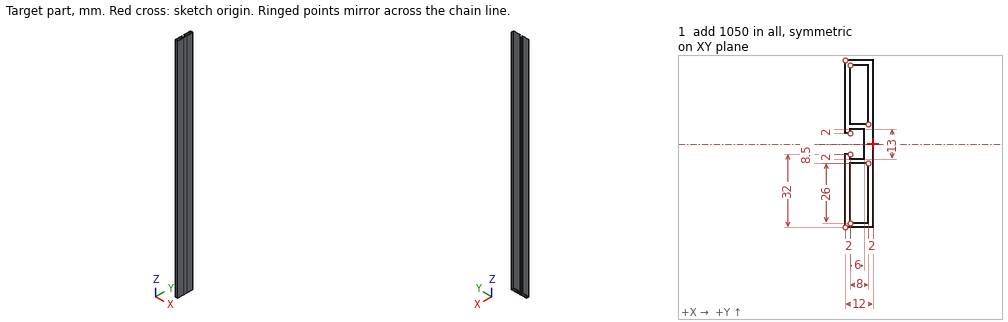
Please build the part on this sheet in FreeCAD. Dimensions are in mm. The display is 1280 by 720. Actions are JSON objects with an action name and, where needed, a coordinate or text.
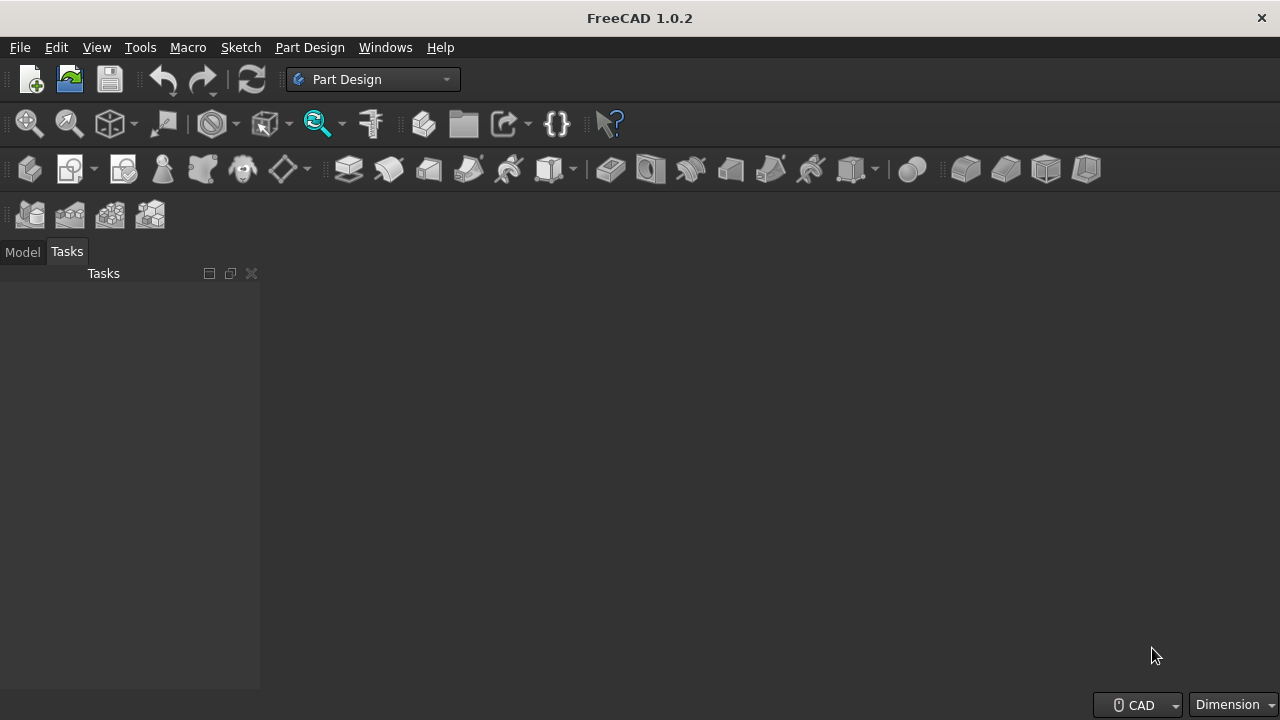
{"action": "left_click", "coordinate": [30, 80]}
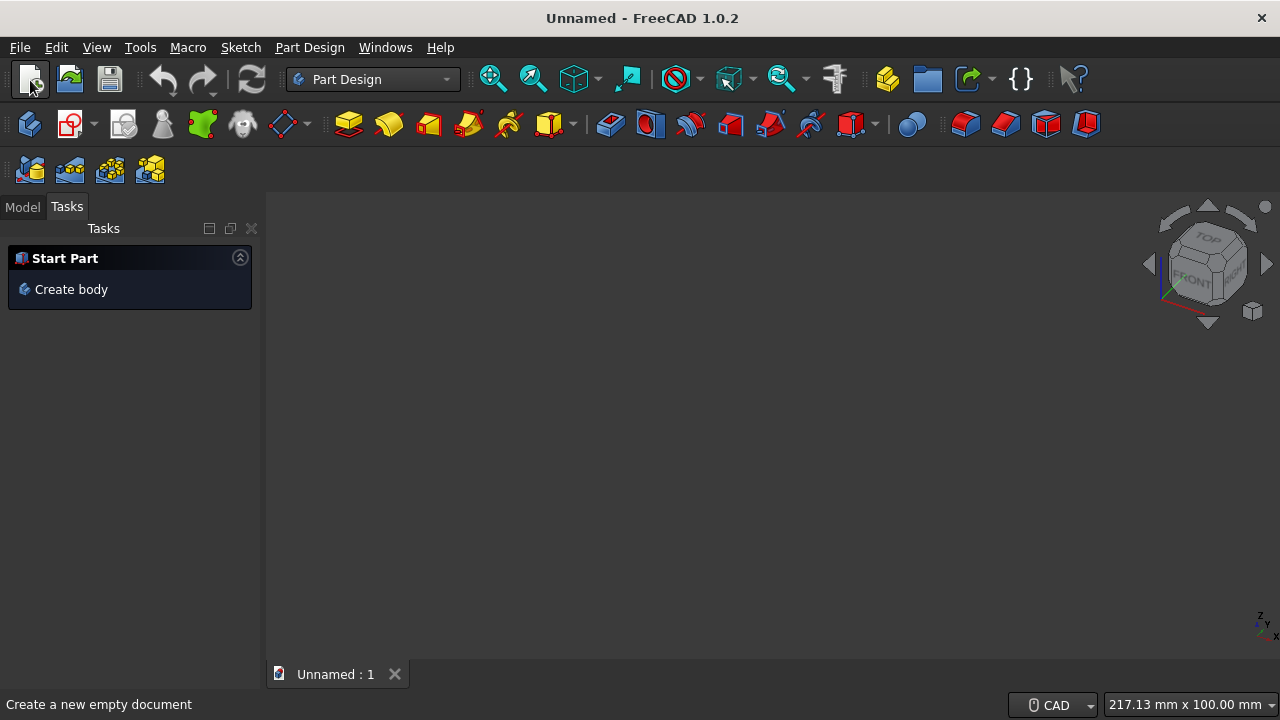
{"action": "left_click", "coordinate": [70, 124]}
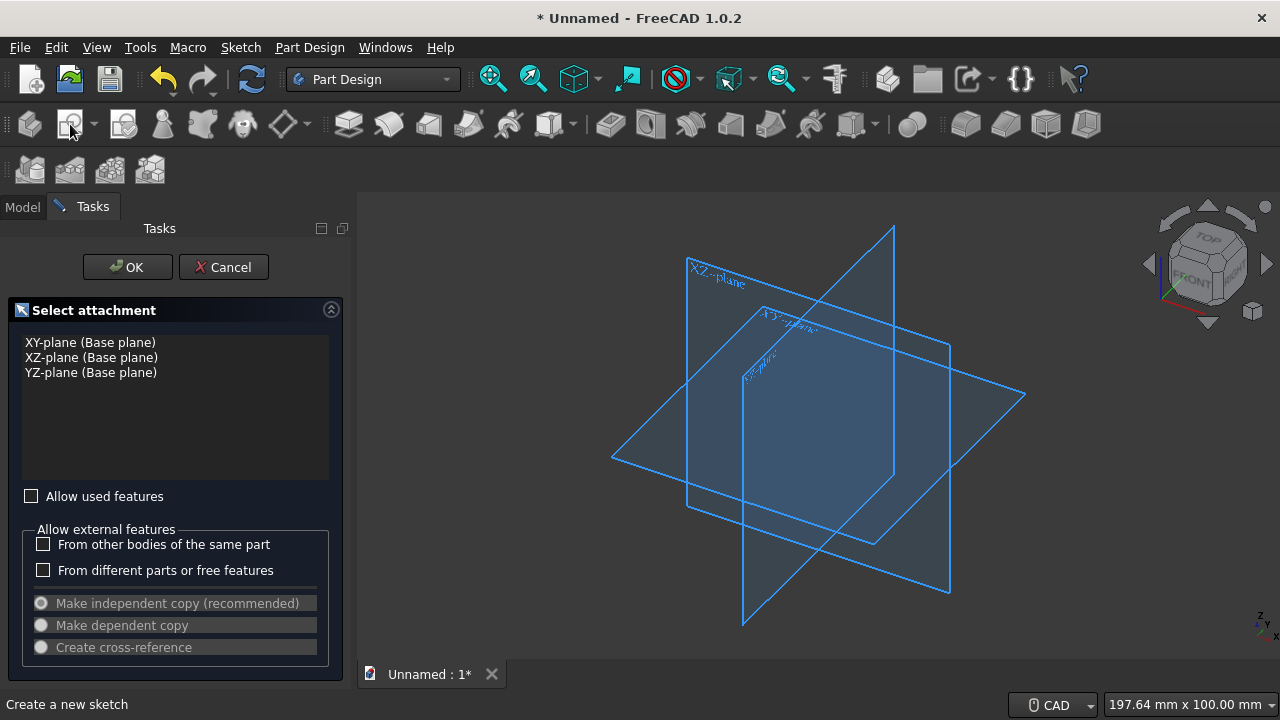
{"action": "left_click", "coordinate": [82, 342]}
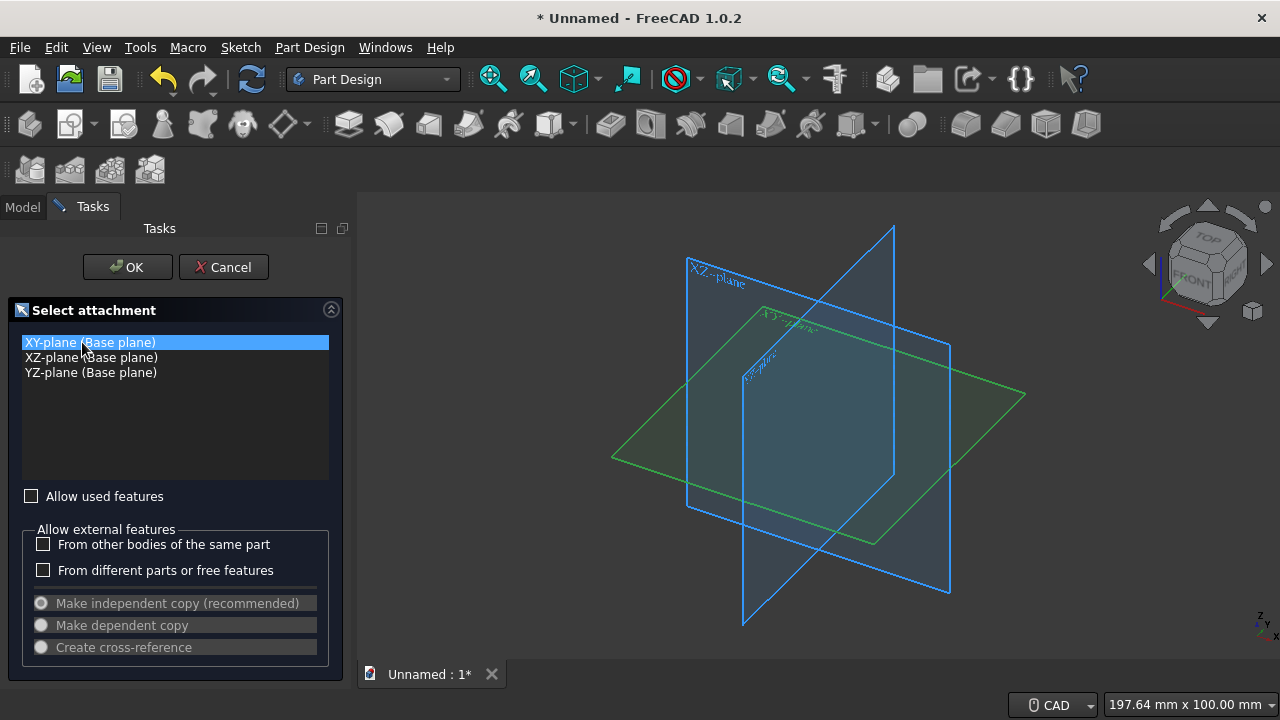
{"action": "left_click", "coordinate": [128, 267]}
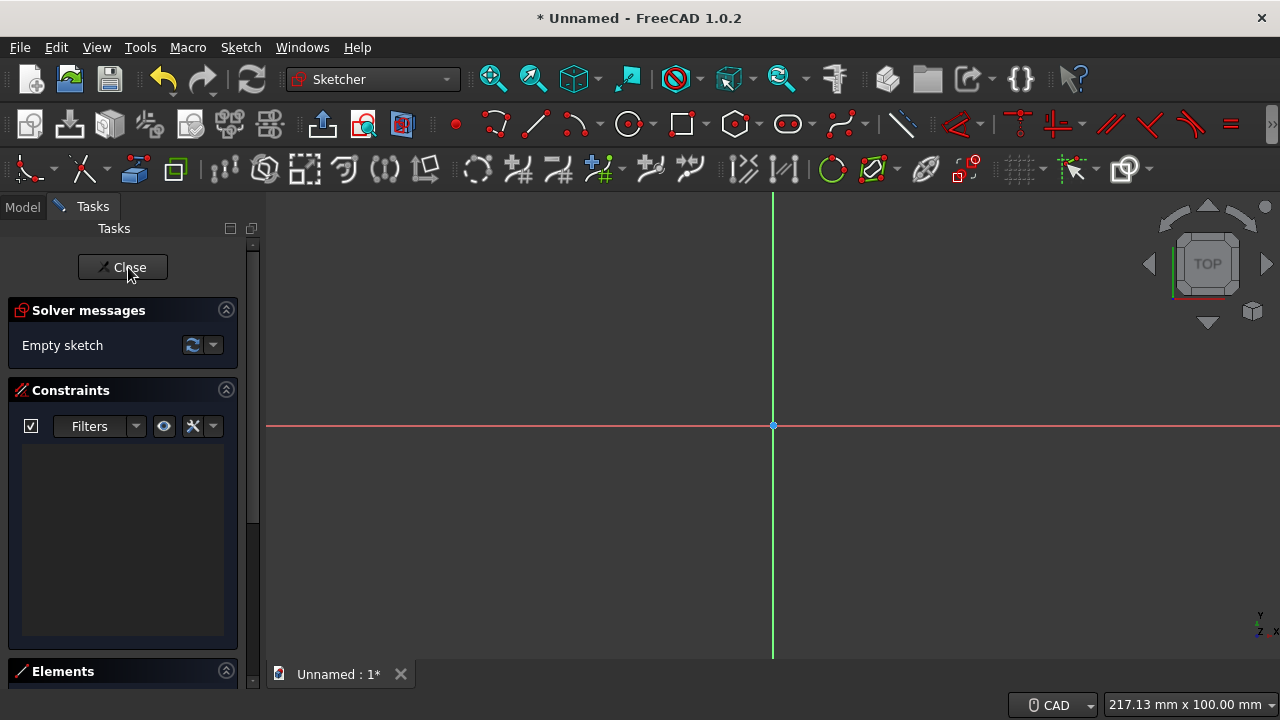
{"action": "left_click", "coordinate": [496, 124]}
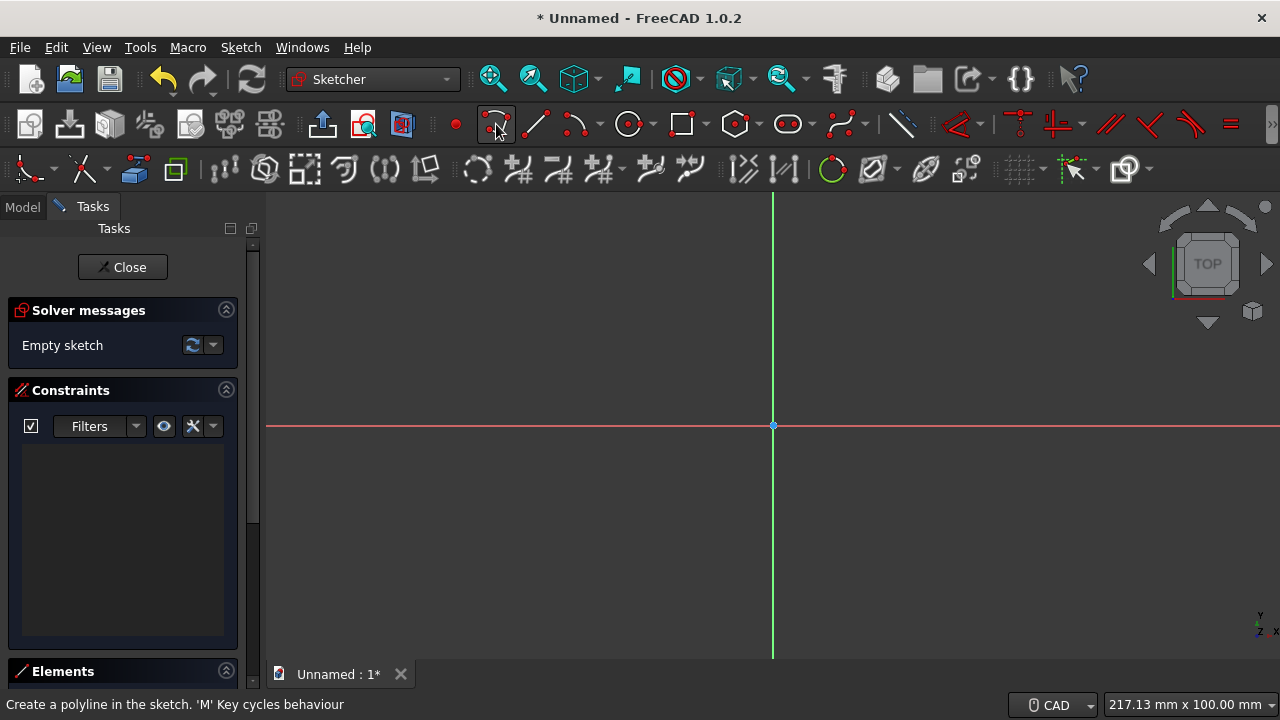
{"action": "left_click", "coordinate": [754, 395]}
{"action": "left_click", "coordinate": [754, 456]}
{"action": "left_click", "coordinate": [726, 456]}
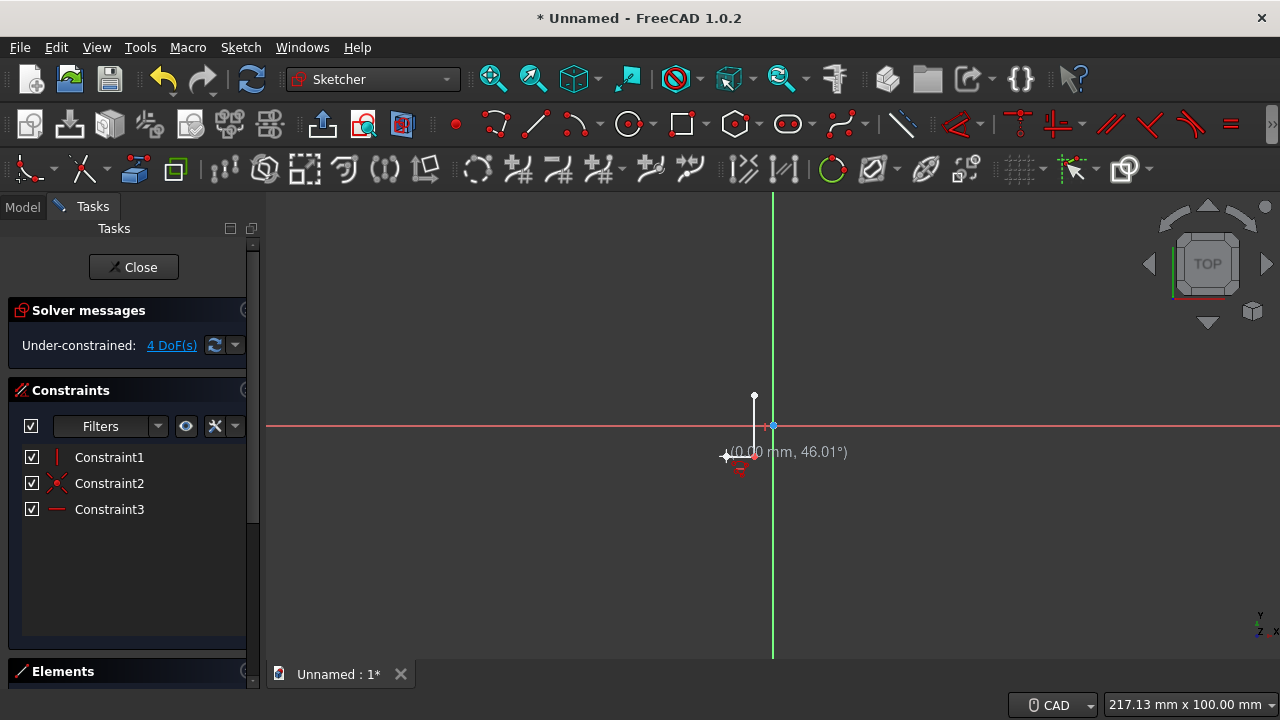
{"action": "scroll", "coordinate": [726, 447], "scroll_direction": "up", "scroll_amount": 3}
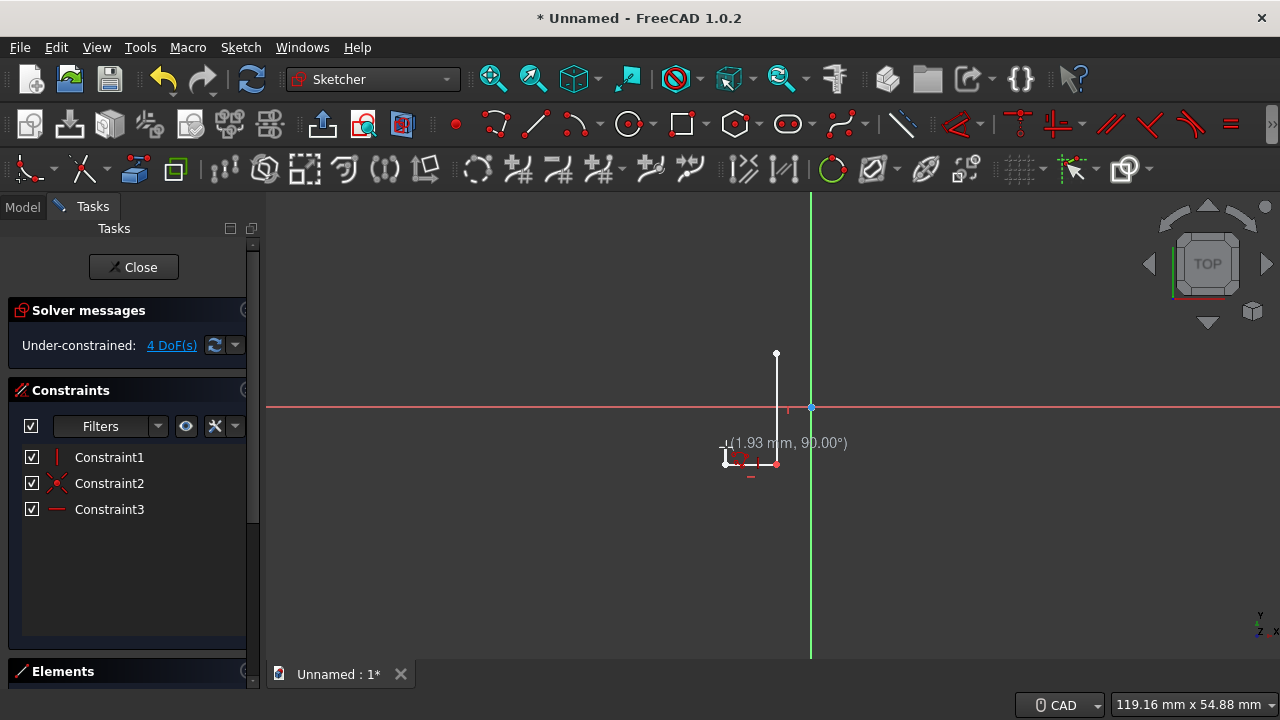
{"action": "left_click", "coordinate": [726, 446]}
{"action": "left_click", "coordinate": [709, 446]}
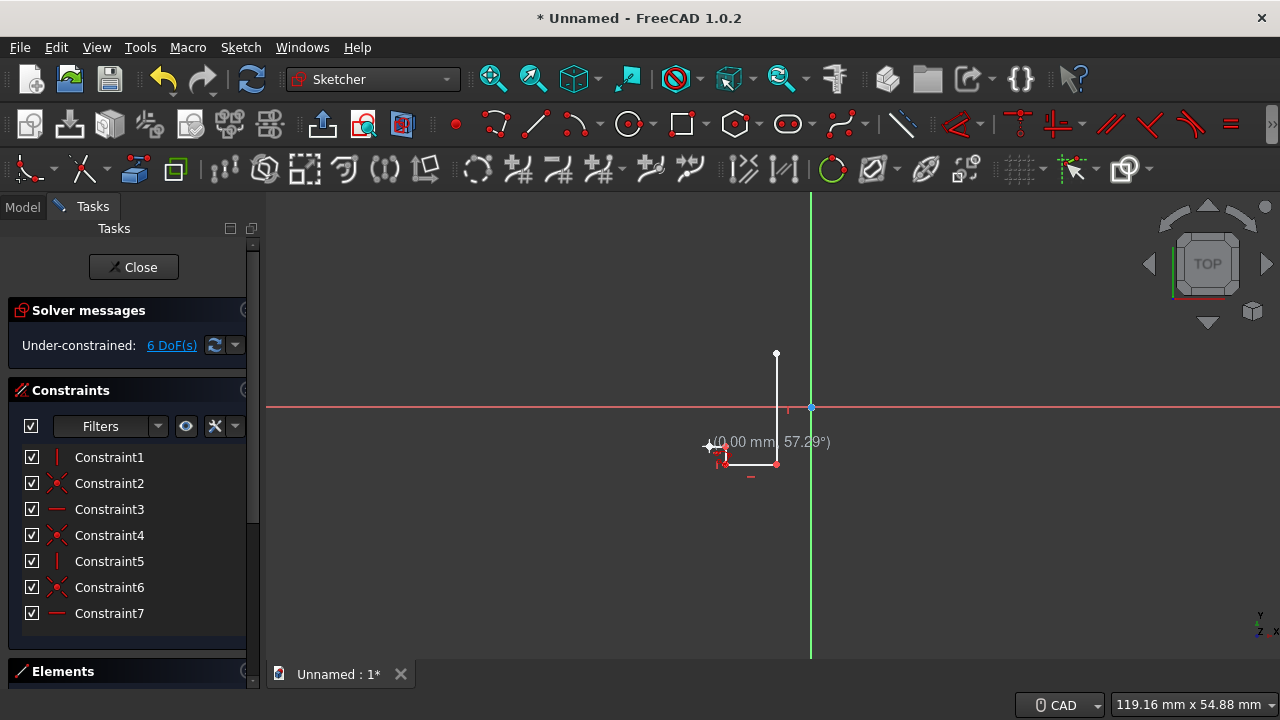
{"action": "scroll", "coordinate": [659, 440], "scroll_direction": "down", "scroll_amount": 4}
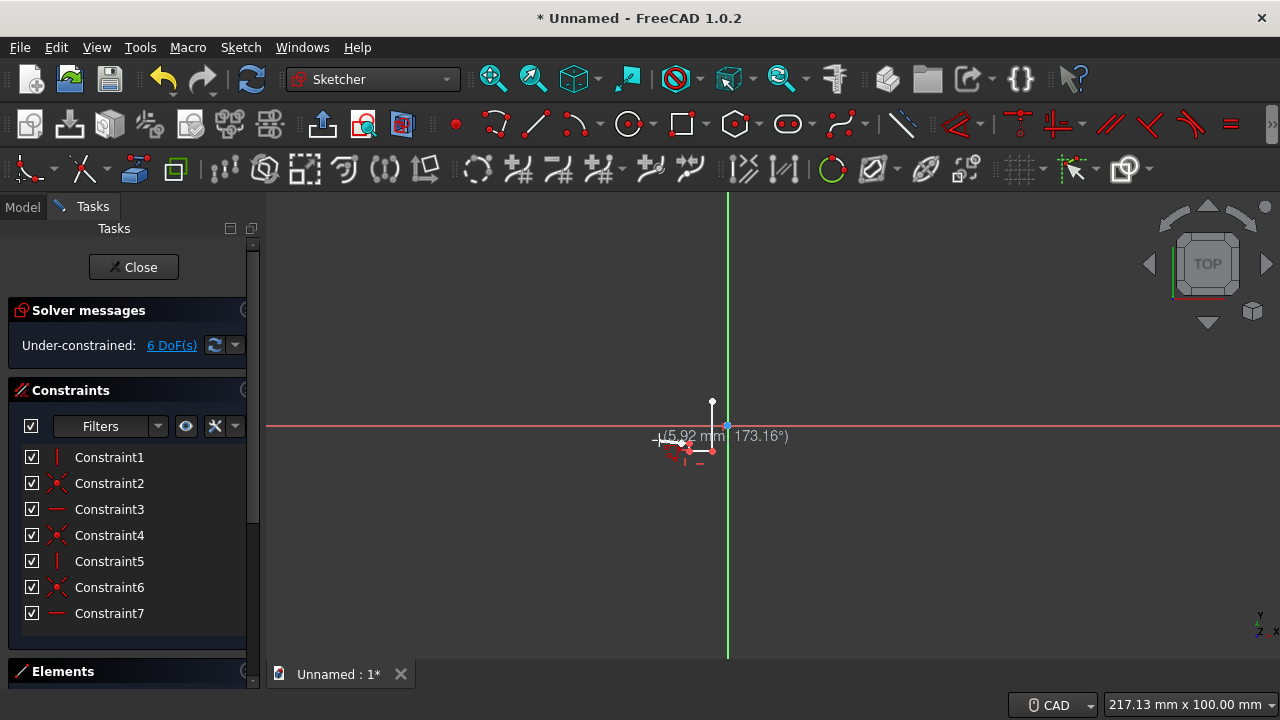
{"action": "left_click", "coordinate": [682, 565]}
{"action": "left_click", "coordinate": [728, 565]}
{"action": "left_click", "coordinate": [719, 286]}
{"action": "left_click", "coordinate": [682, 286]}
{"action": "left_click", "coordinate": [682, 408]}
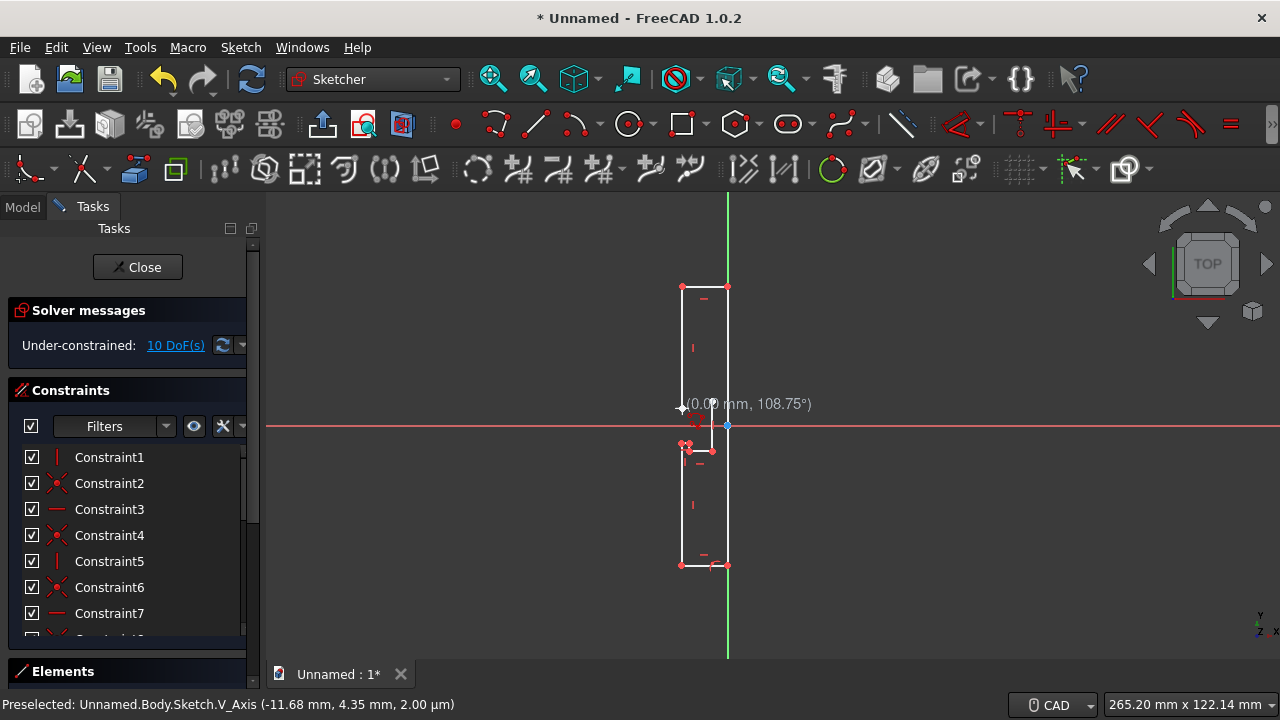
{"action": "scroll", "coordinate": [689, 408], "scroll_direction": "up", "scroll_amount": 4}